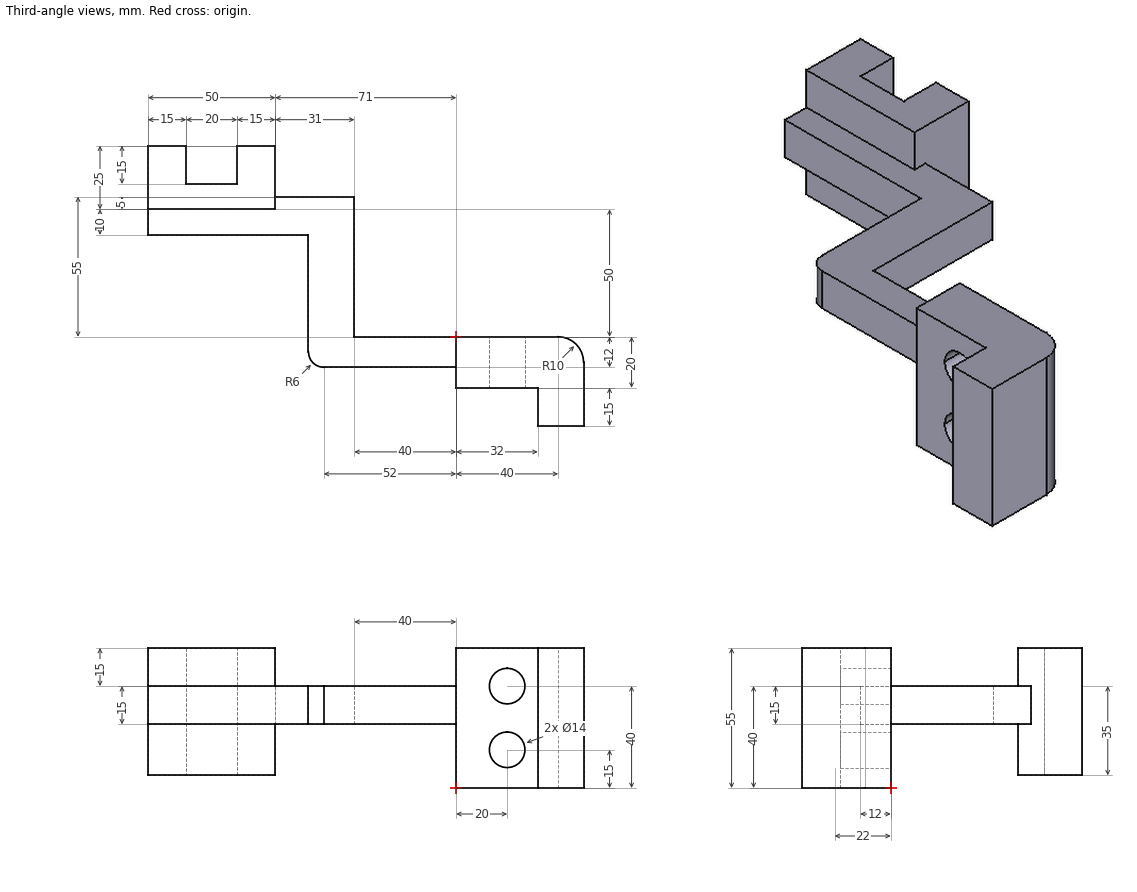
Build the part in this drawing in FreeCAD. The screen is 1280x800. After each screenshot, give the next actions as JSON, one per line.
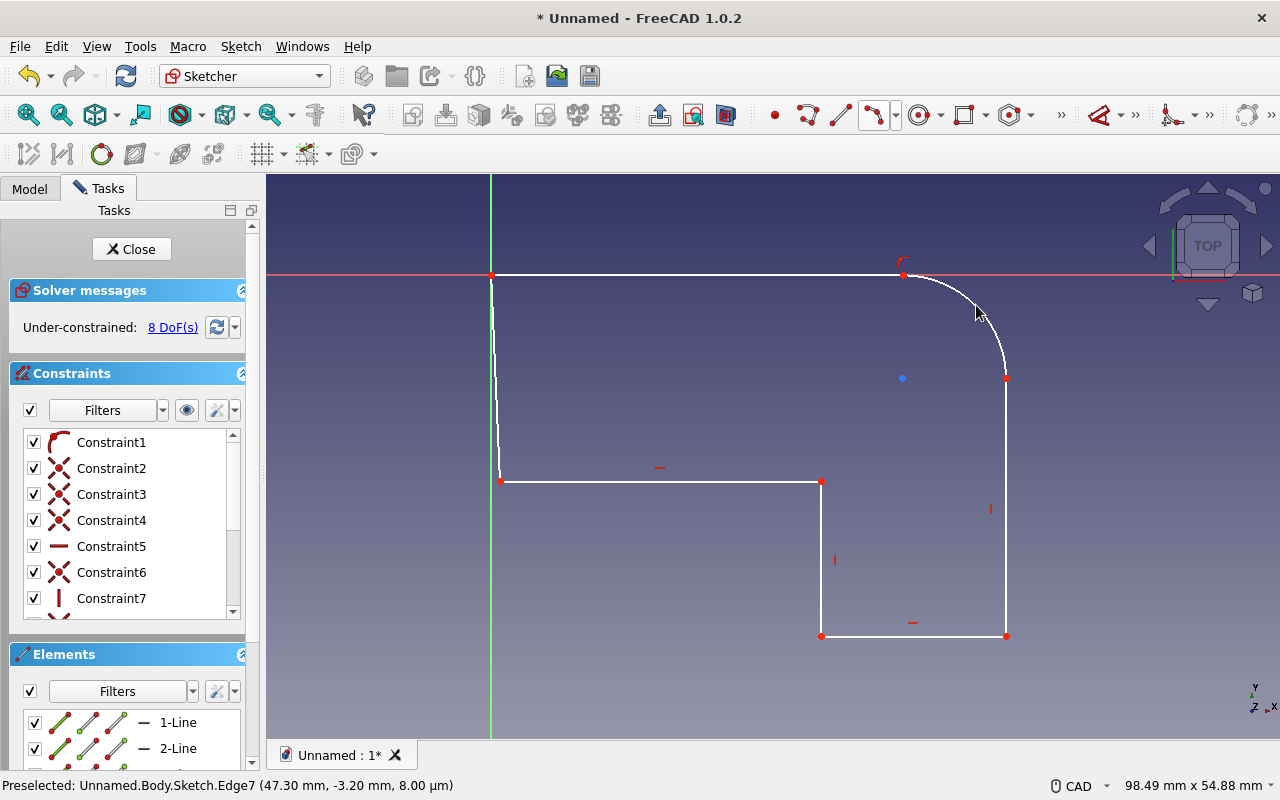
{"action": "left_click", "coordinate": [779, 275]}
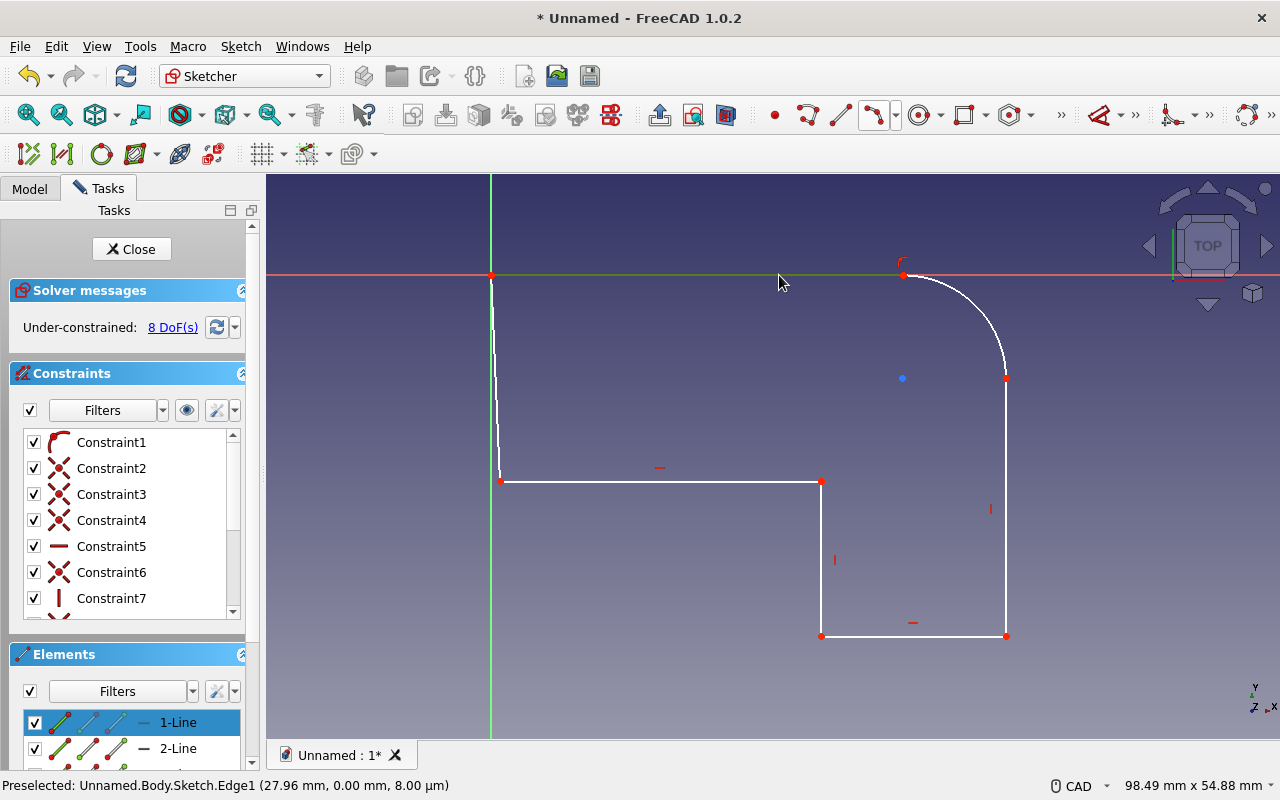
{"action": "left_click", "coordinate": [995, 332]}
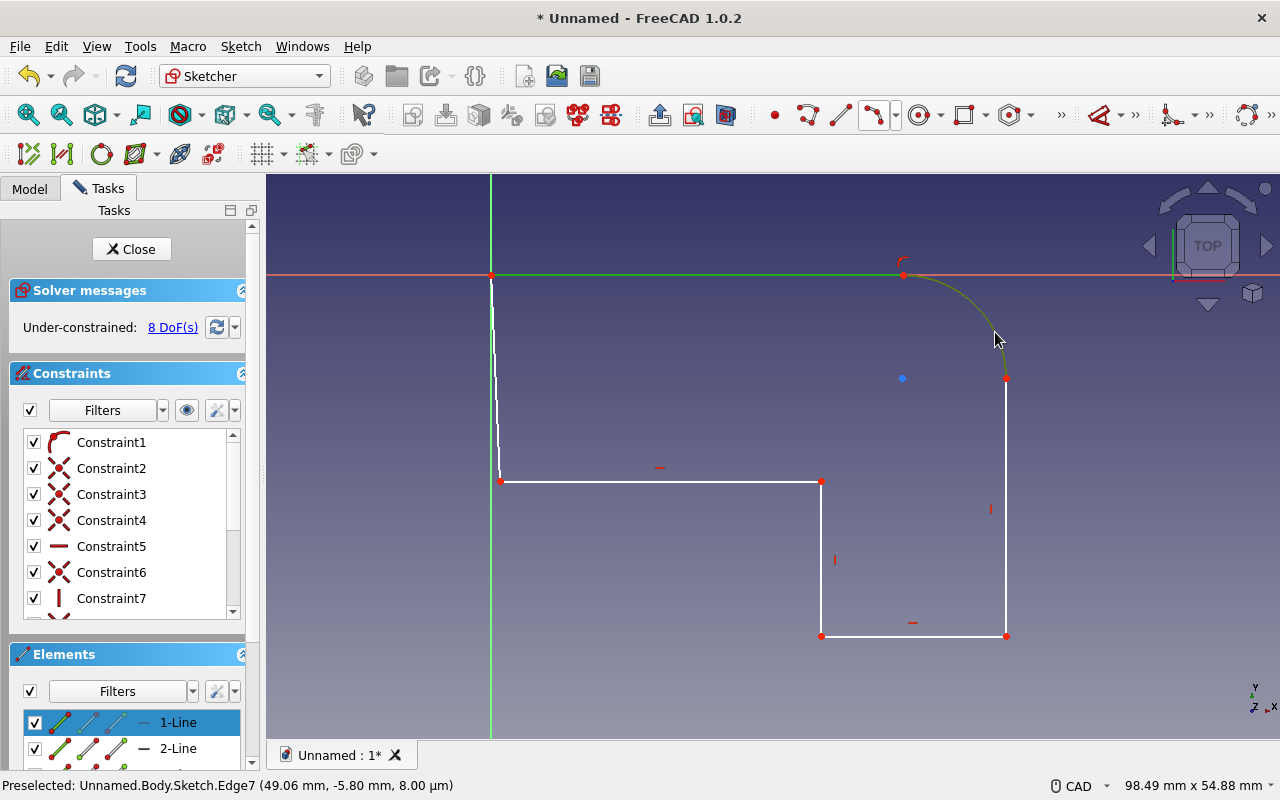
{"action": "key", "text": "t"}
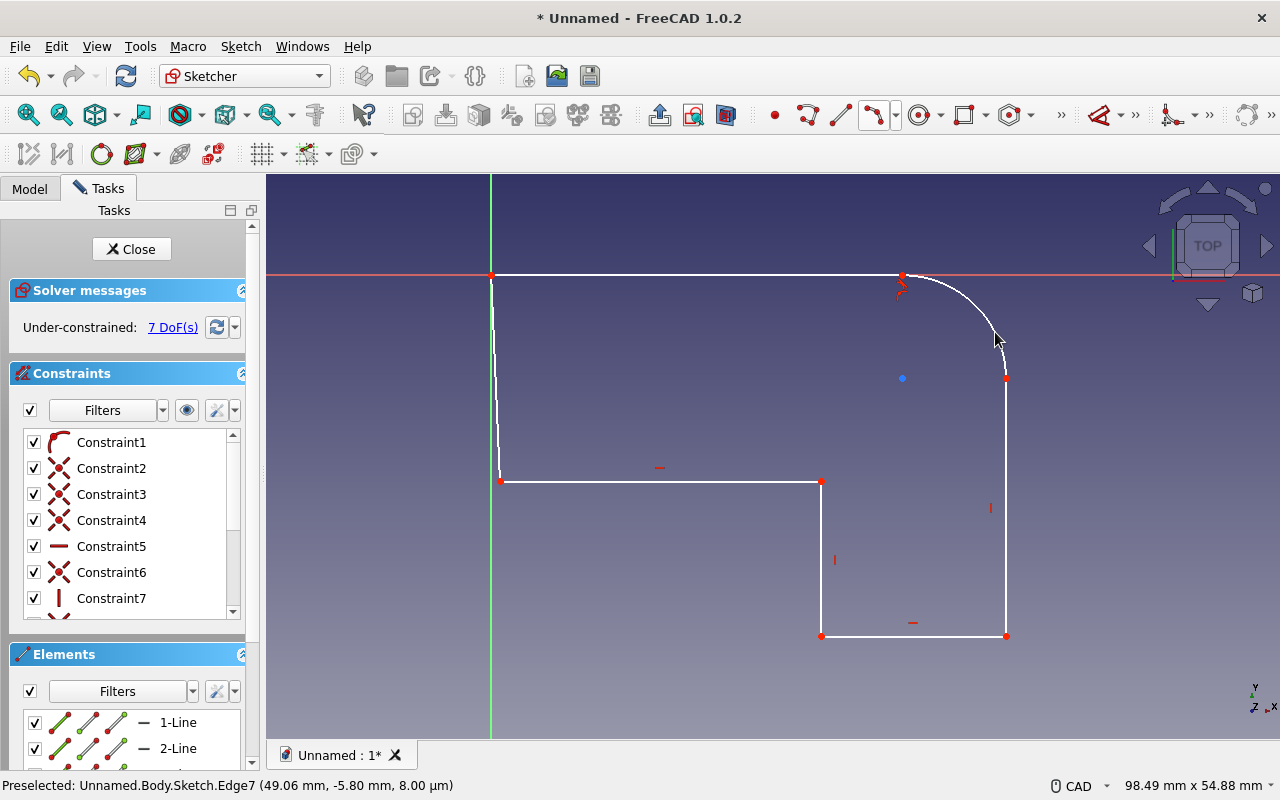
{"action": "left_click", "coordinate": [1006, 560]}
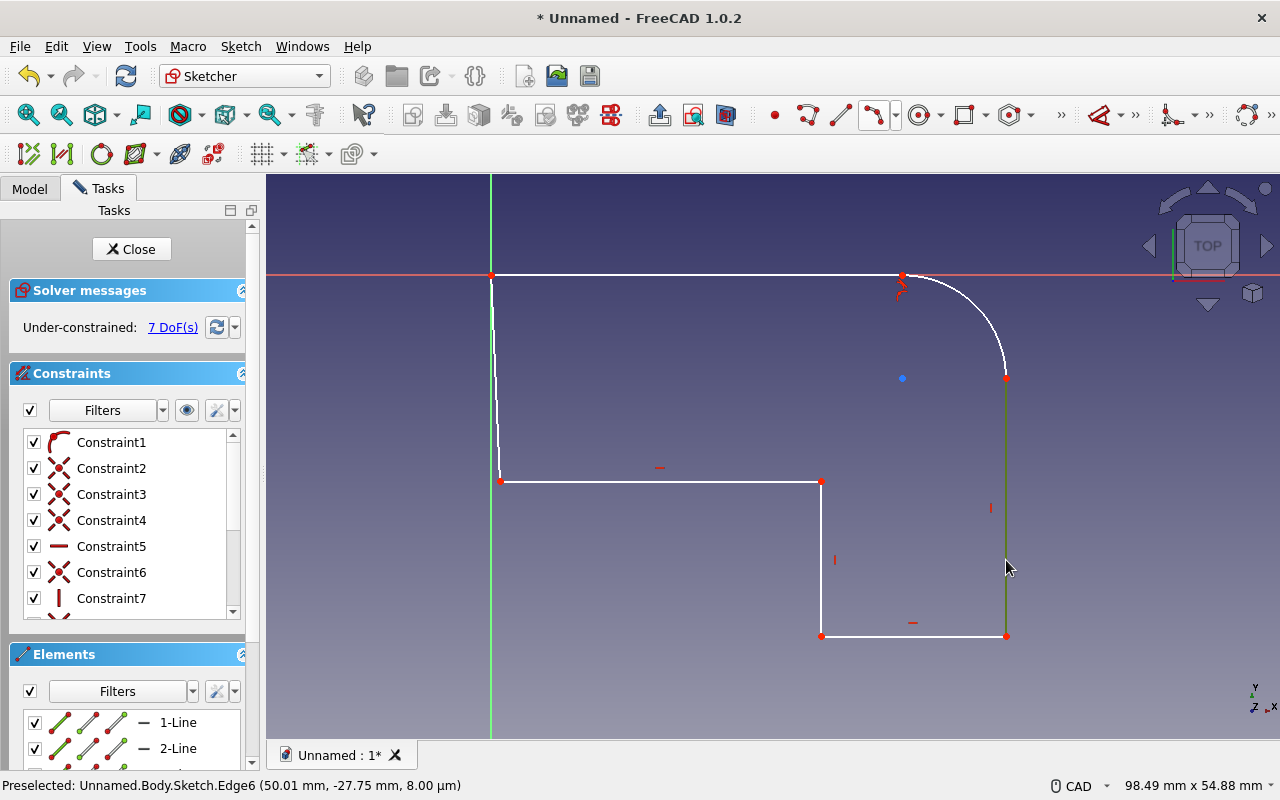
{"action": "left_click", "coordinate": [995, 332]}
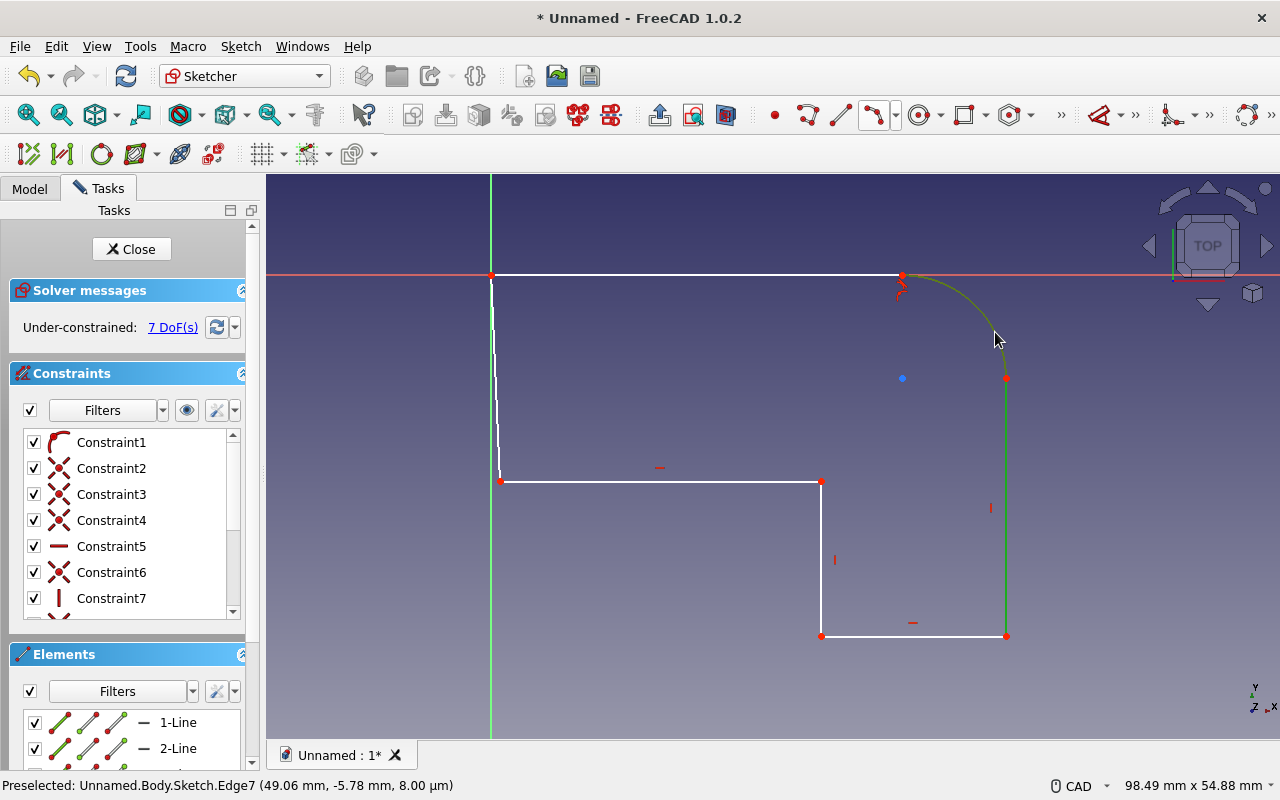
{"action": "key", "text": "t"}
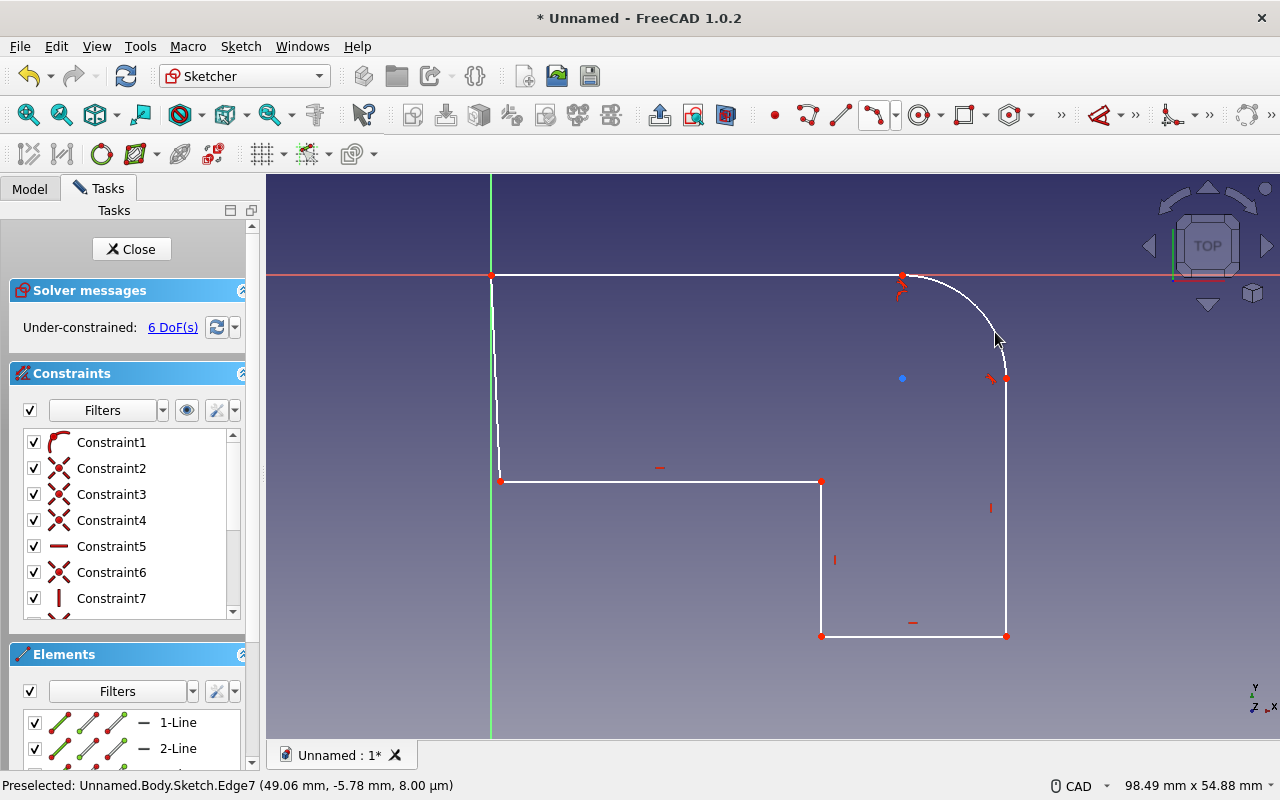
{"action": "left_click", "coordinate": [494, 337]}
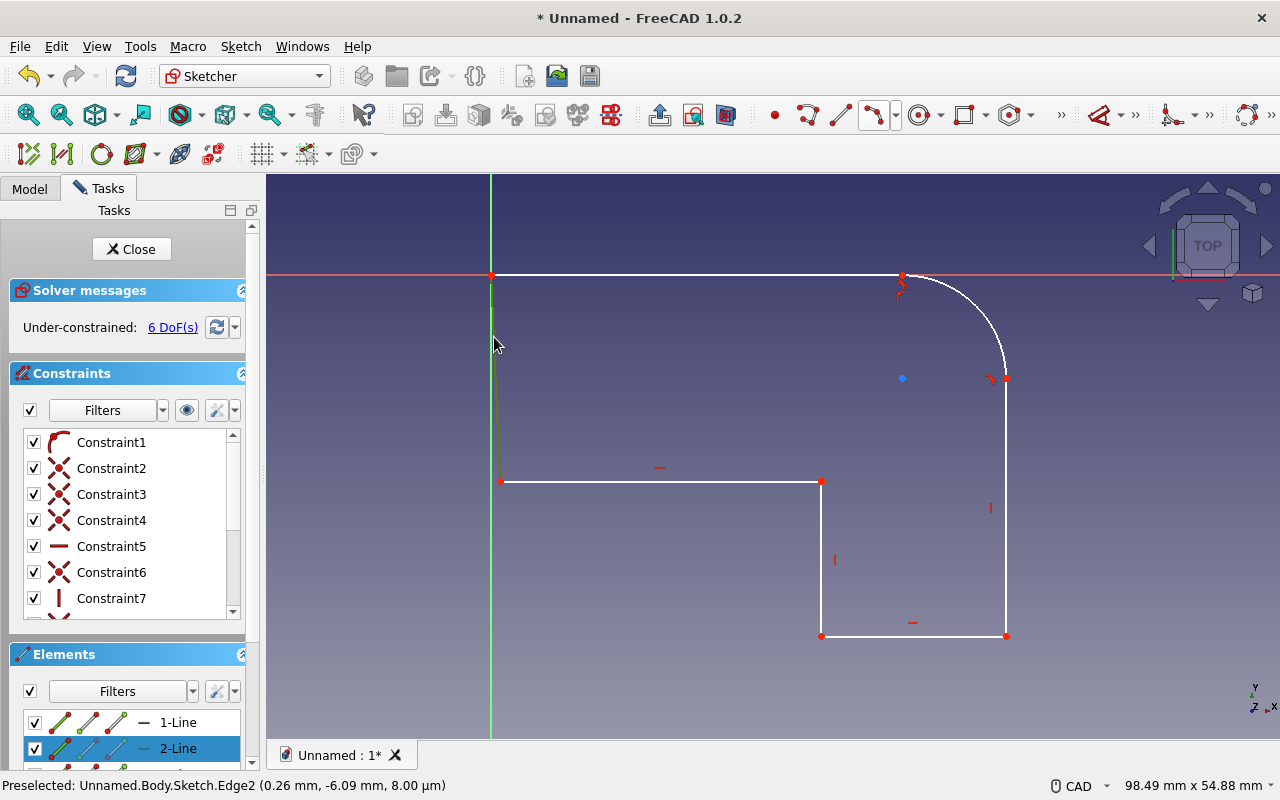
{"action": "key", "text": "v"}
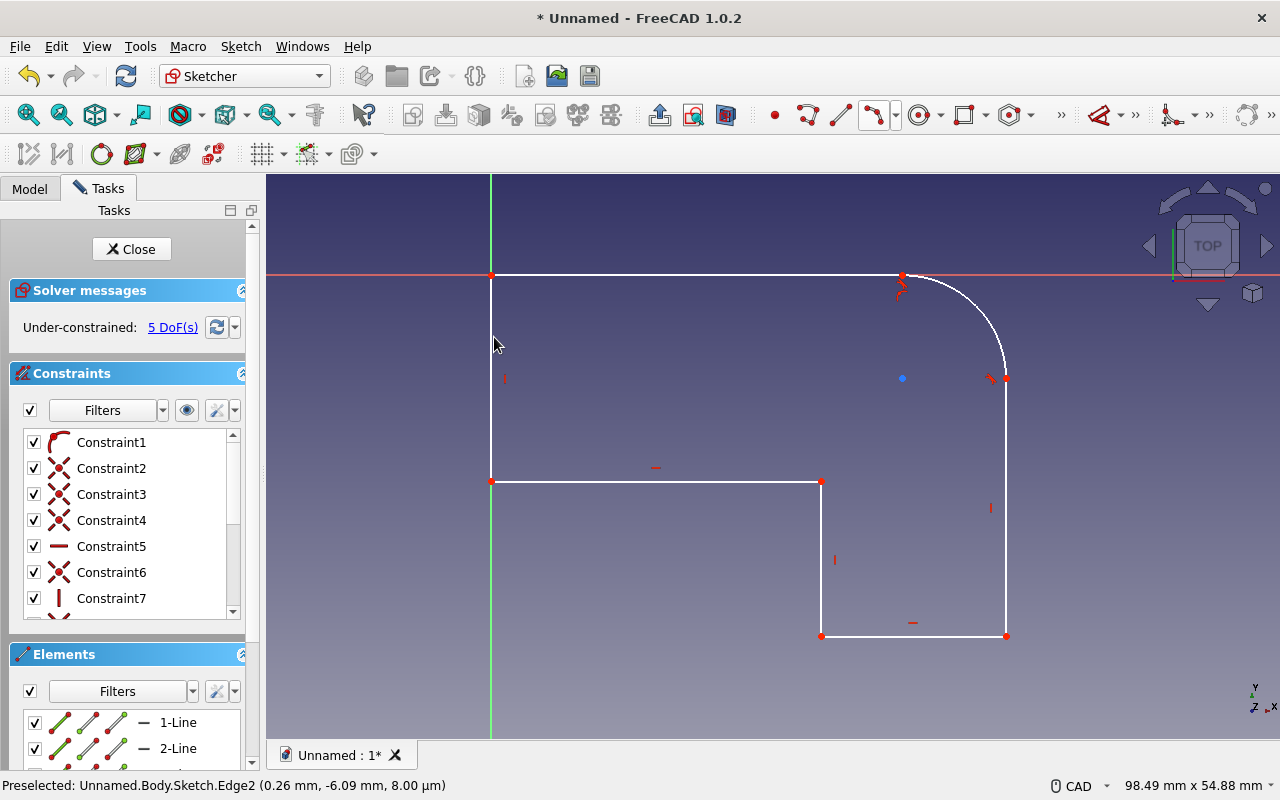
{"action": "left_click", "coordinate": [1098, 116]}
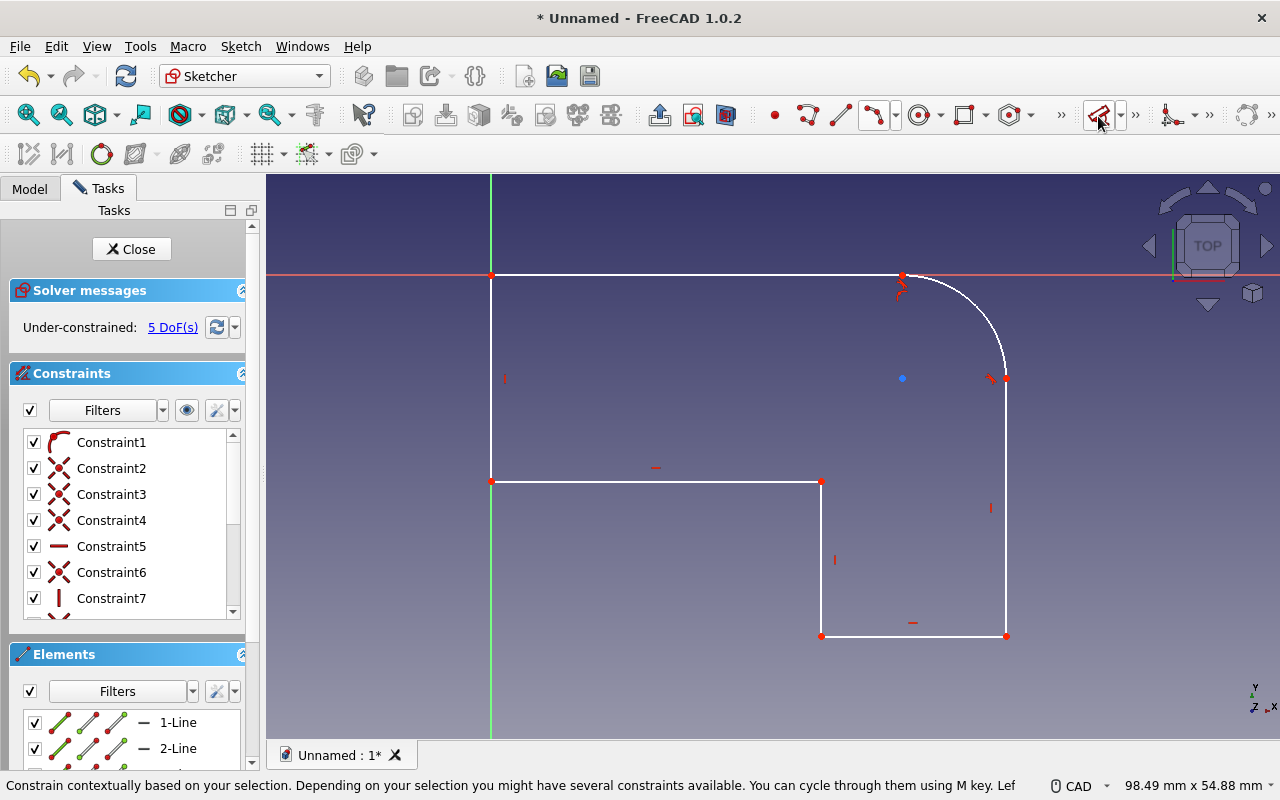
{"action": "left_click", "coordinate": [995, 332]}
{"action": "left_click", "coordinate": [1024, 318]}